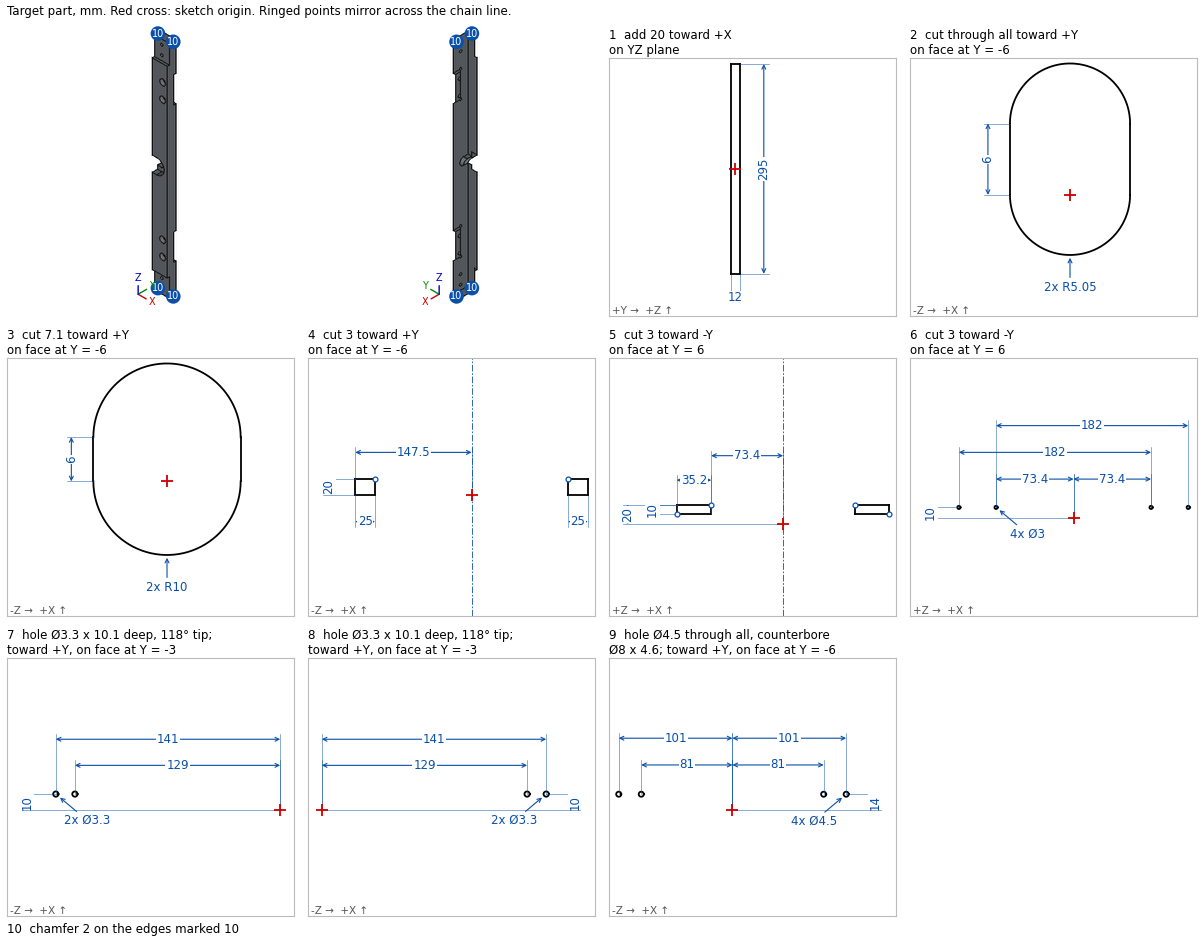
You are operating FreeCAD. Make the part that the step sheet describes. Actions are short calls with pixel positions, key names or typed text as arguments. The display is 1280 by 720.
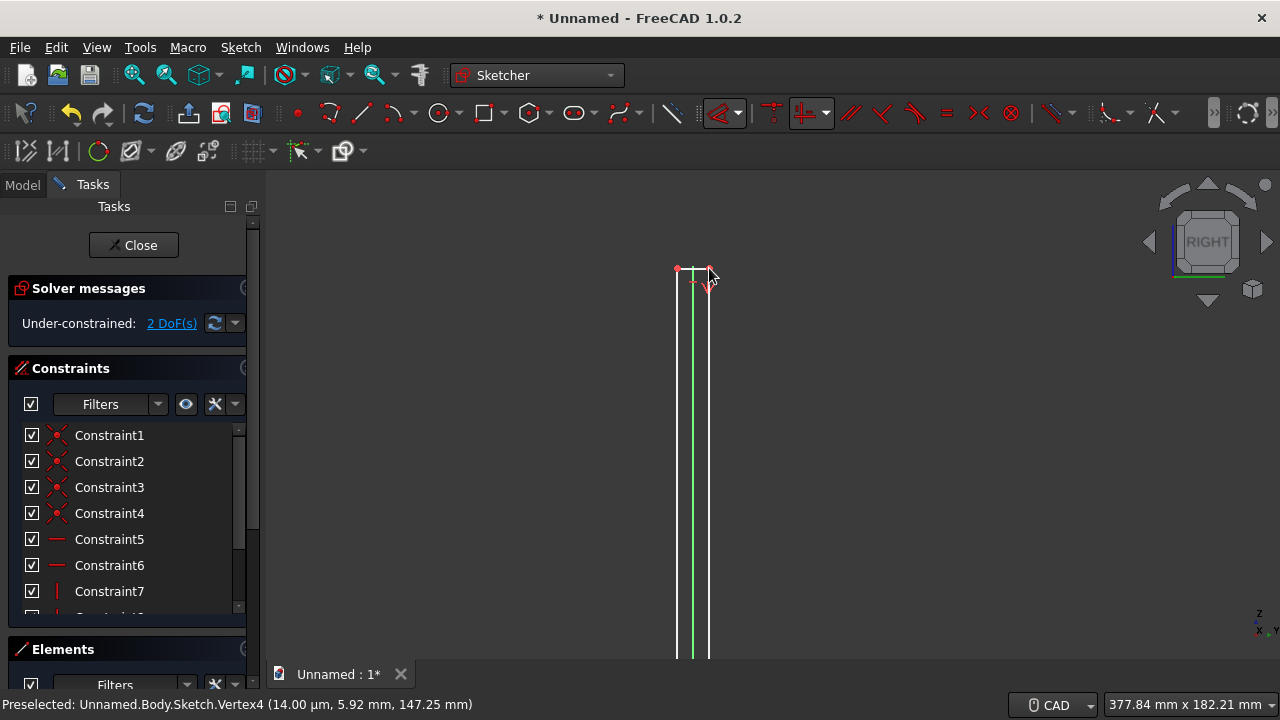
click(718, 114)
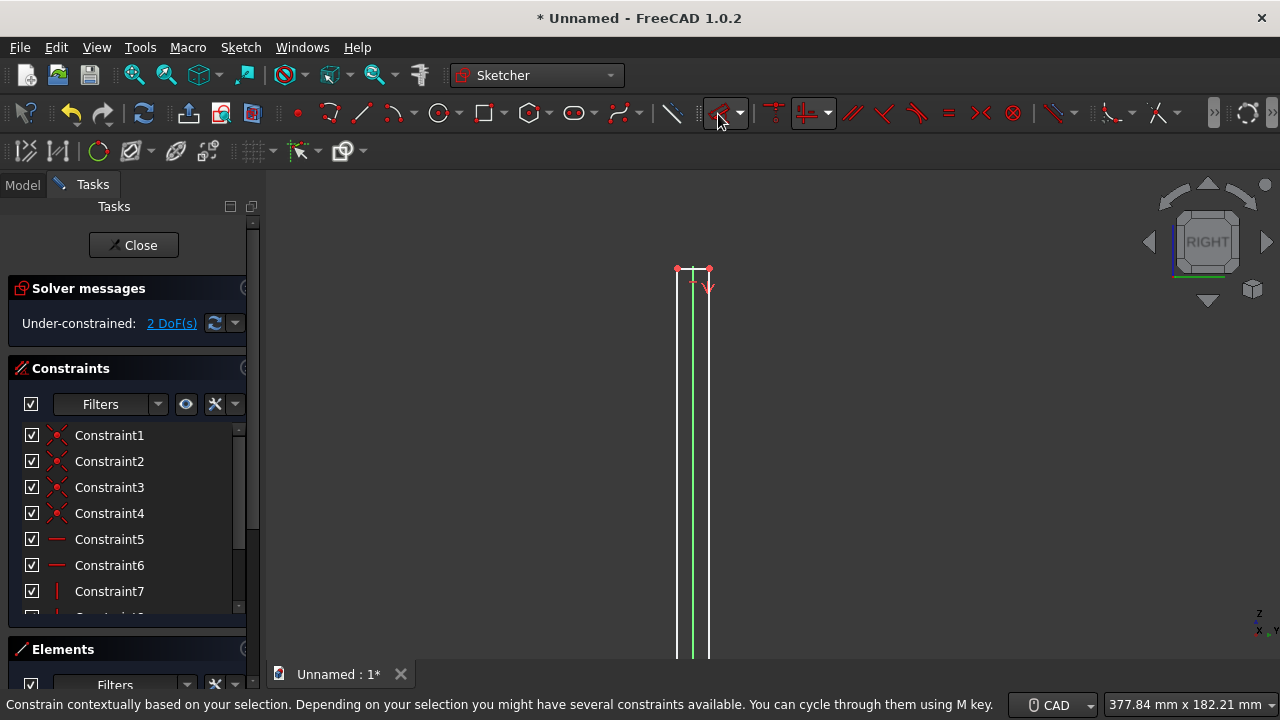
scroll(711, 269, down, 5)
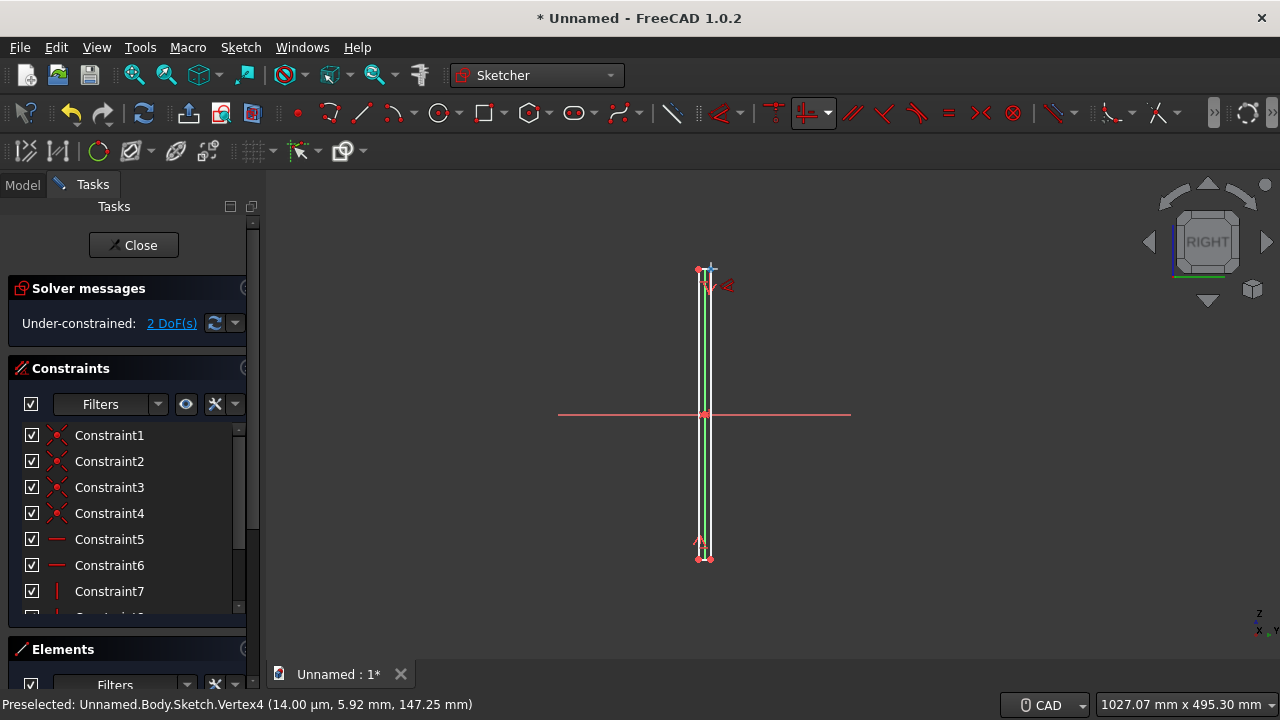
scroll(704, 560, up, 7)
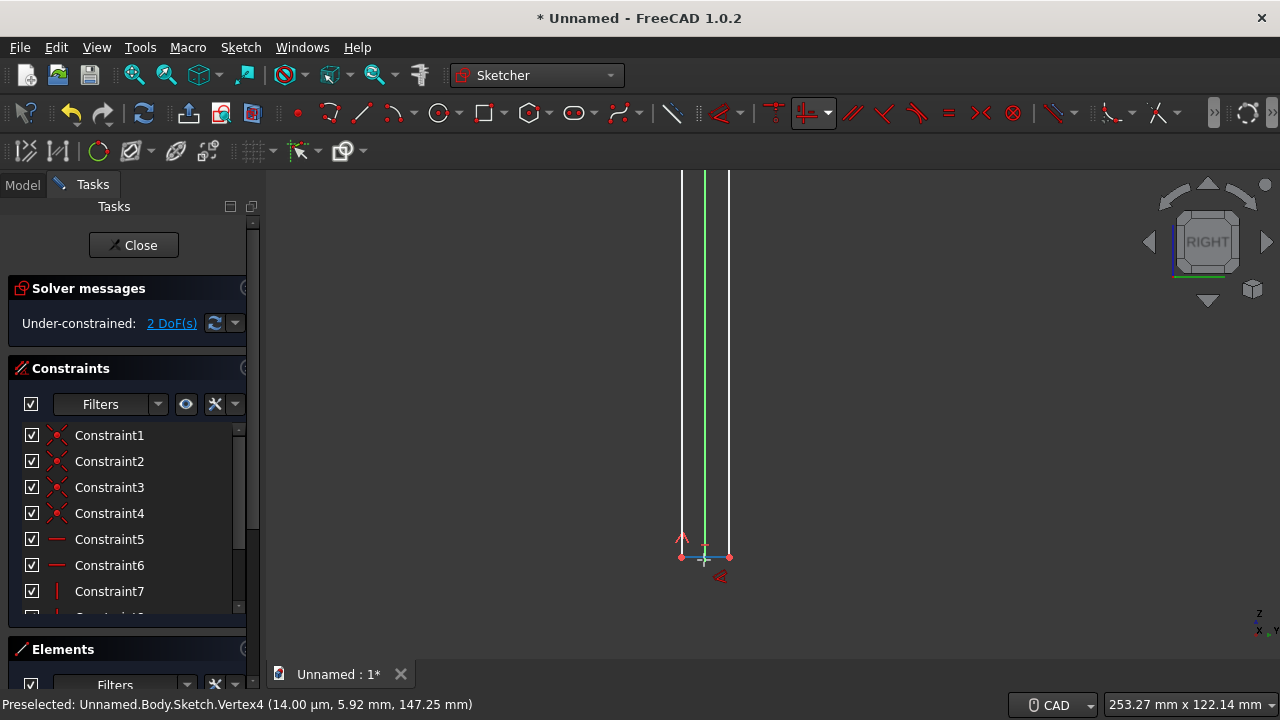
click(701, 557)
click(689, 591)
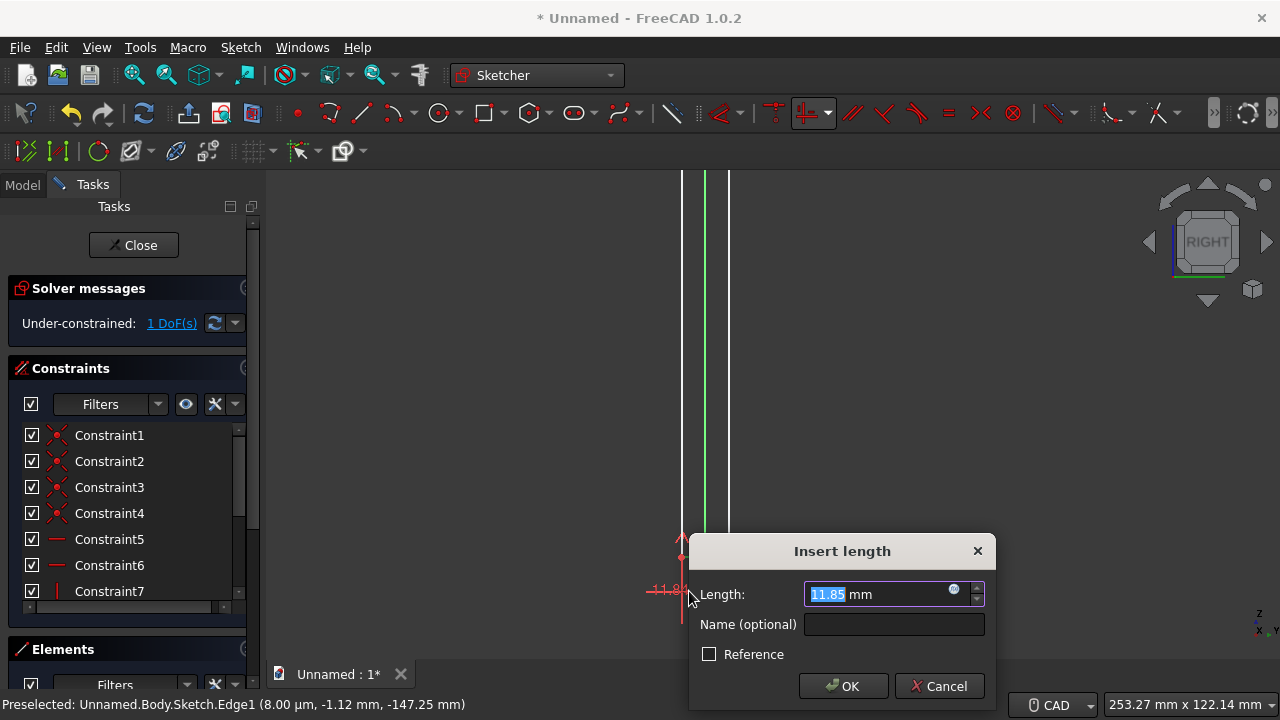
text(12)
key(Return)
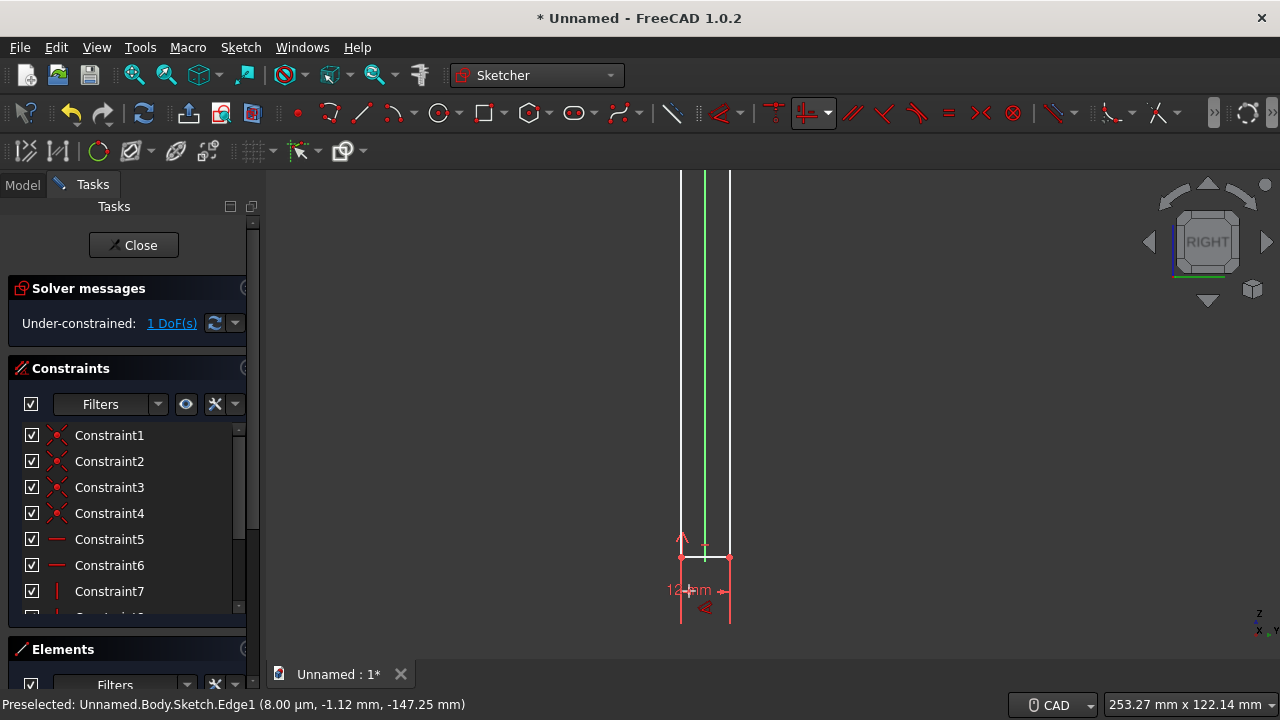
click(730, 203)
click(764, 378)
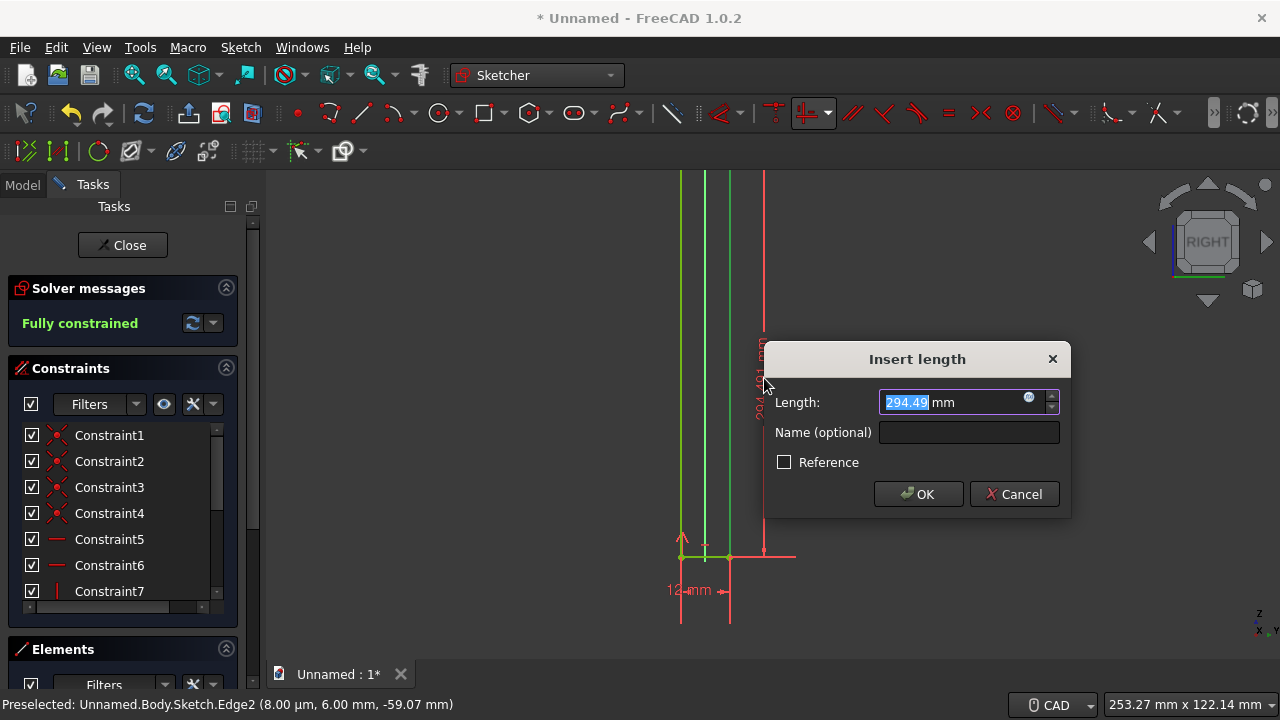
text(295)
key(Return)
key(Escape)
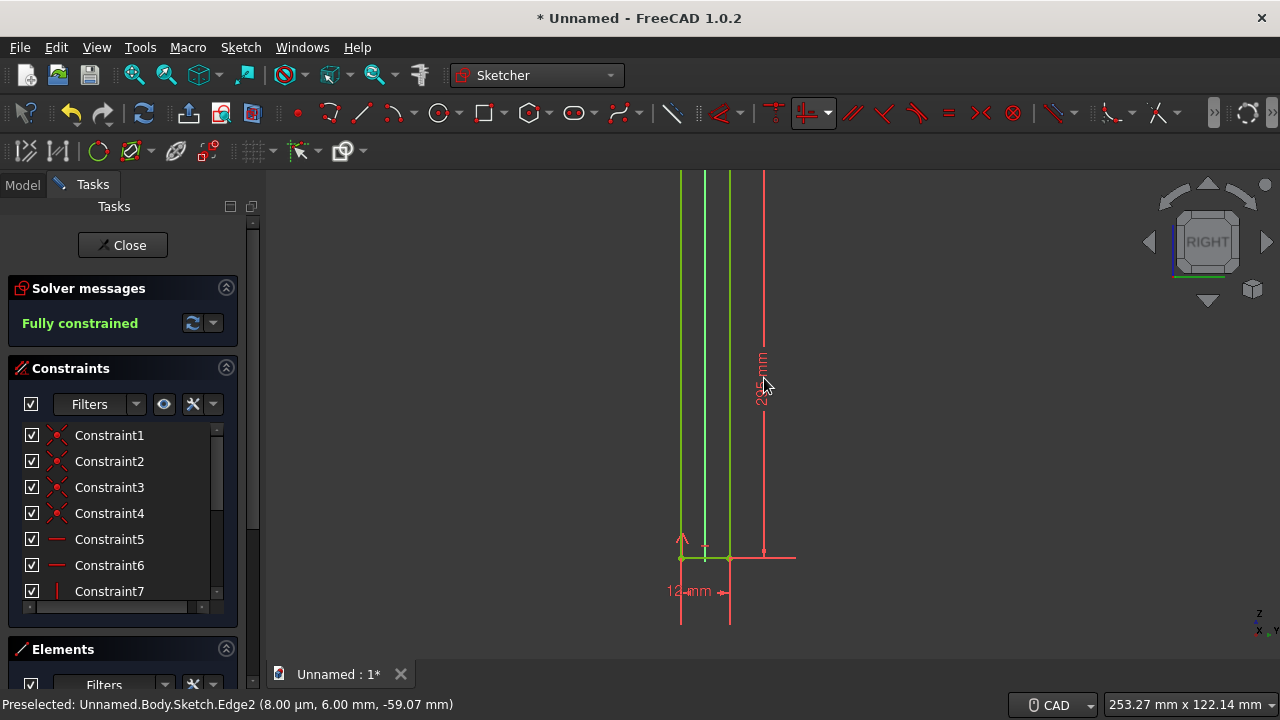
click(123, 245)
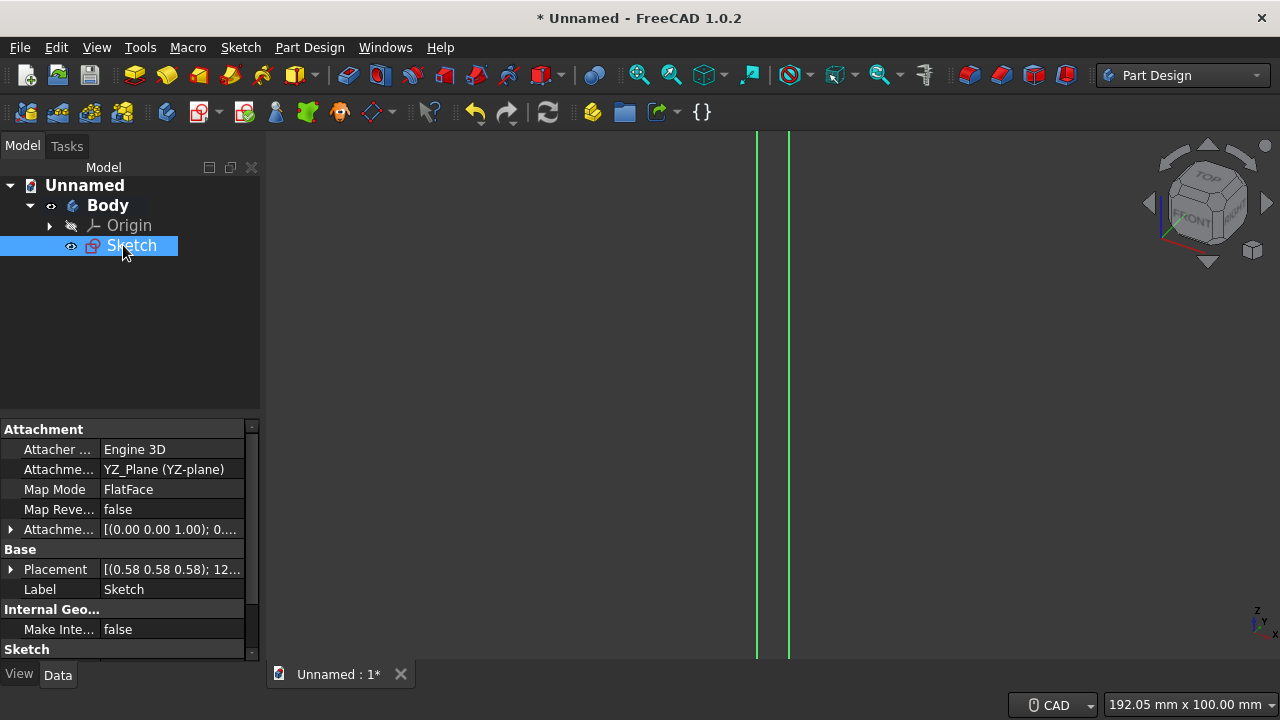
click(136, 76)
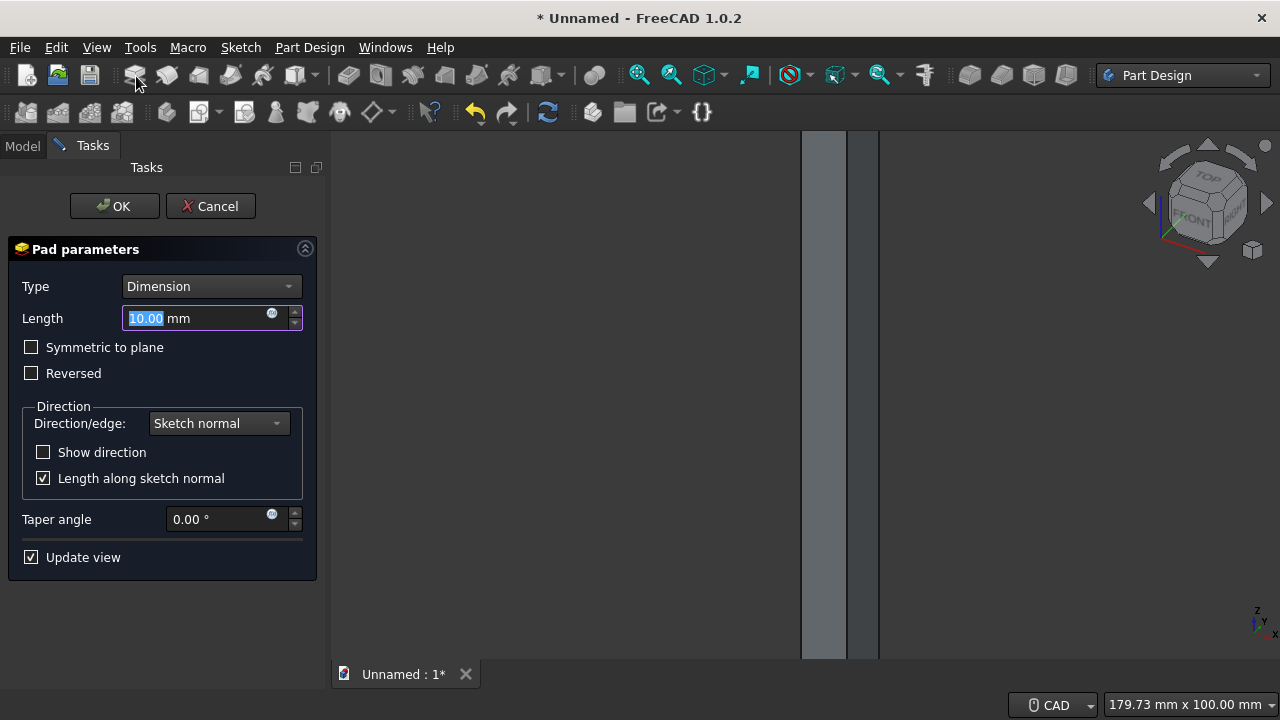
text(20)
key(Tab)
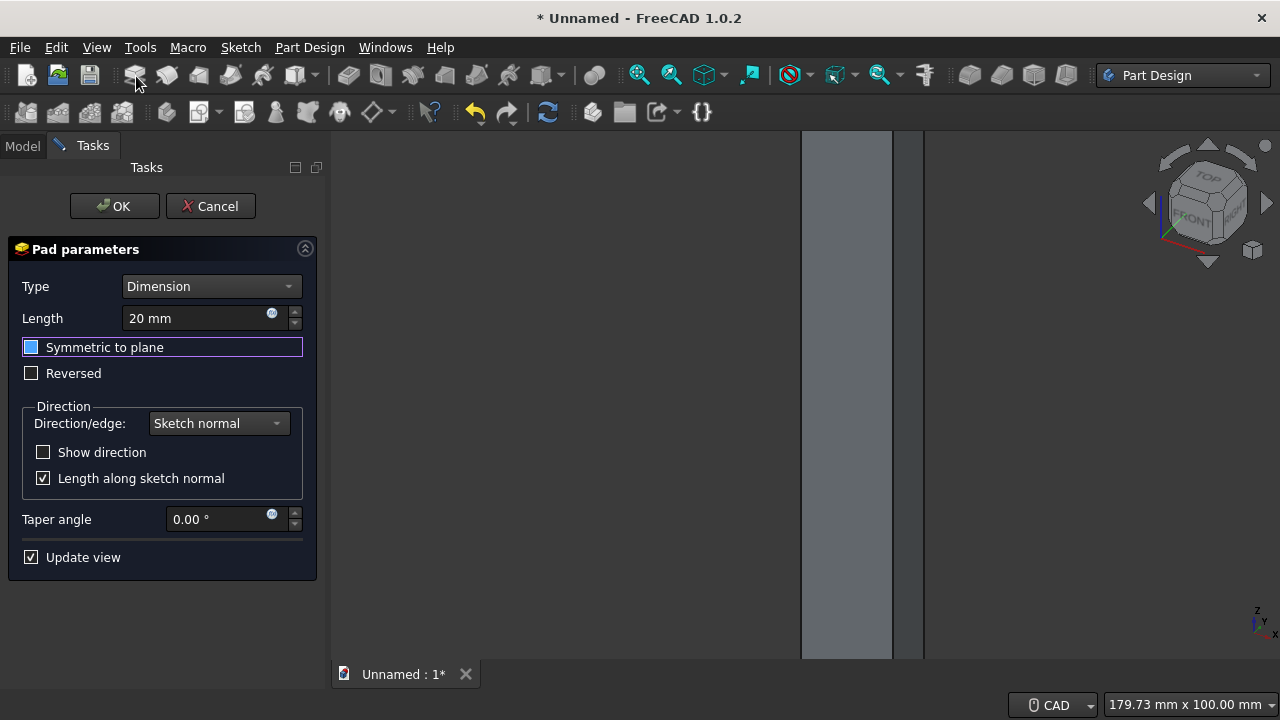
click(115, 206)